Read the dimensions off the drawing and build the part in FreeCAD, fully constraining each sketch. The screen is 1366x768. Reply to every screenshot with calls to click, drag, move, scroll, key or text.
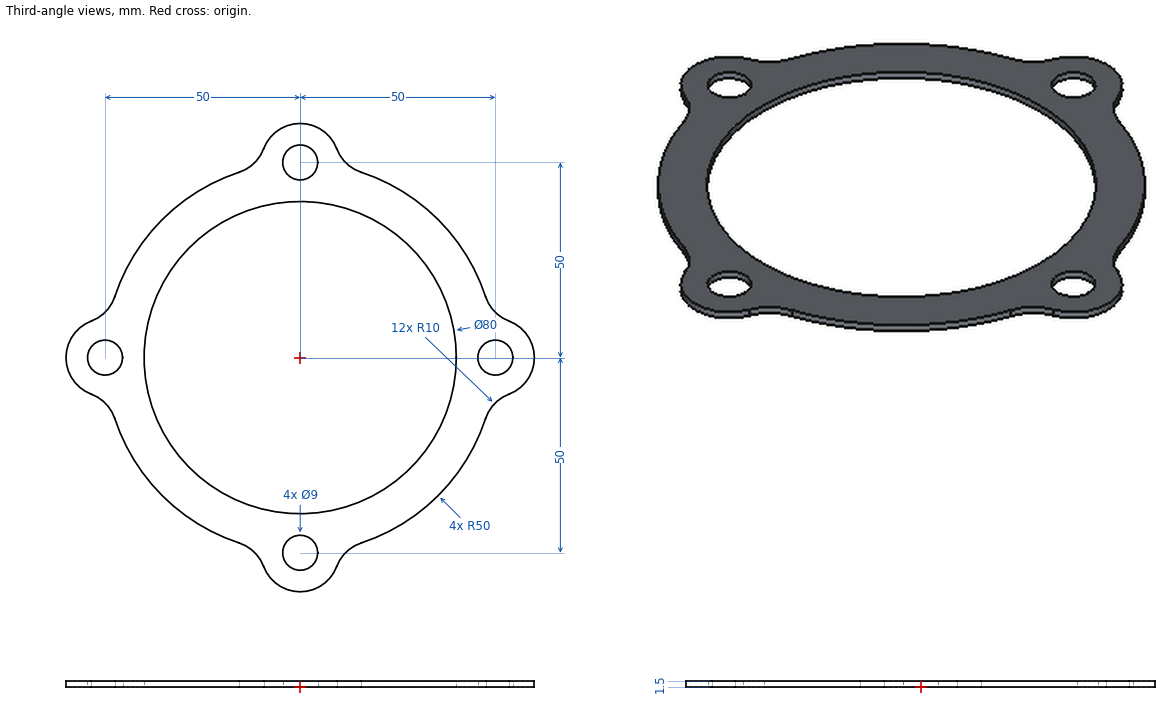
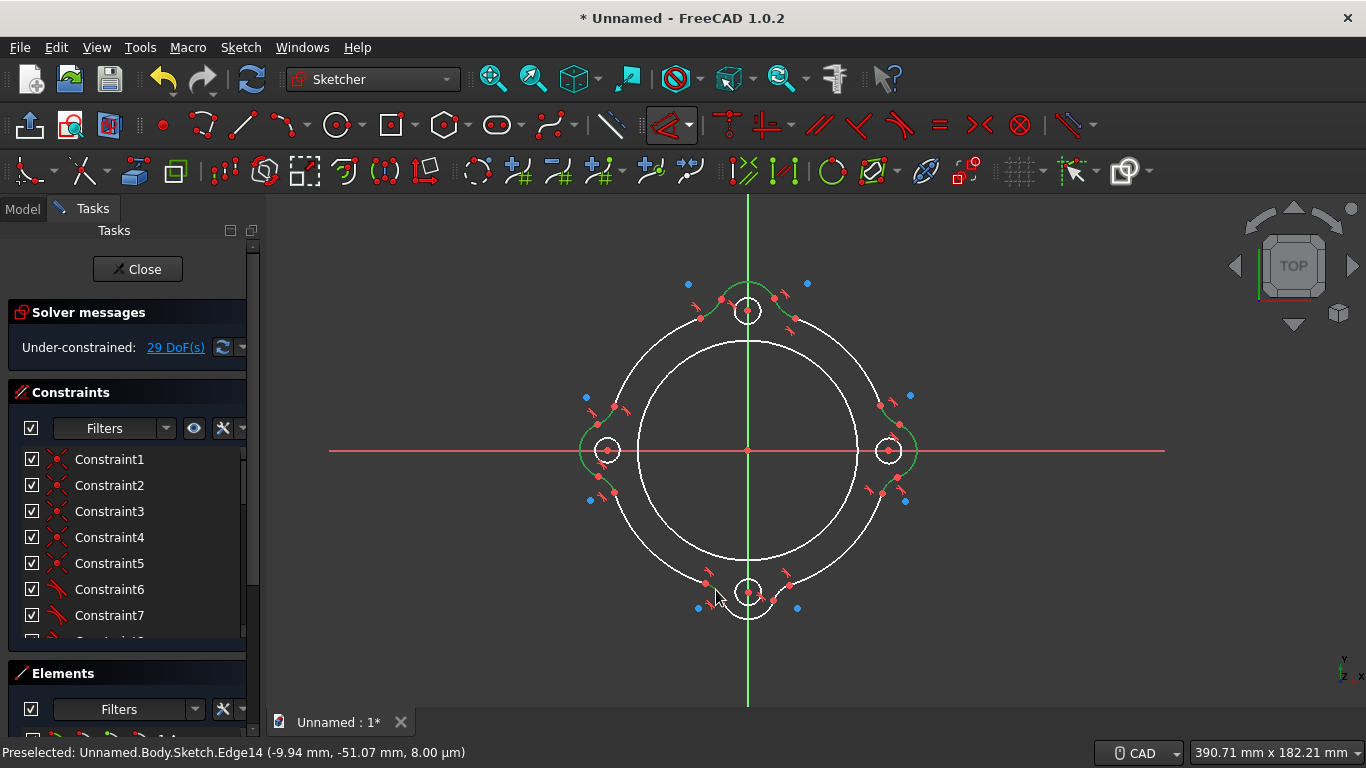
click(735, 616)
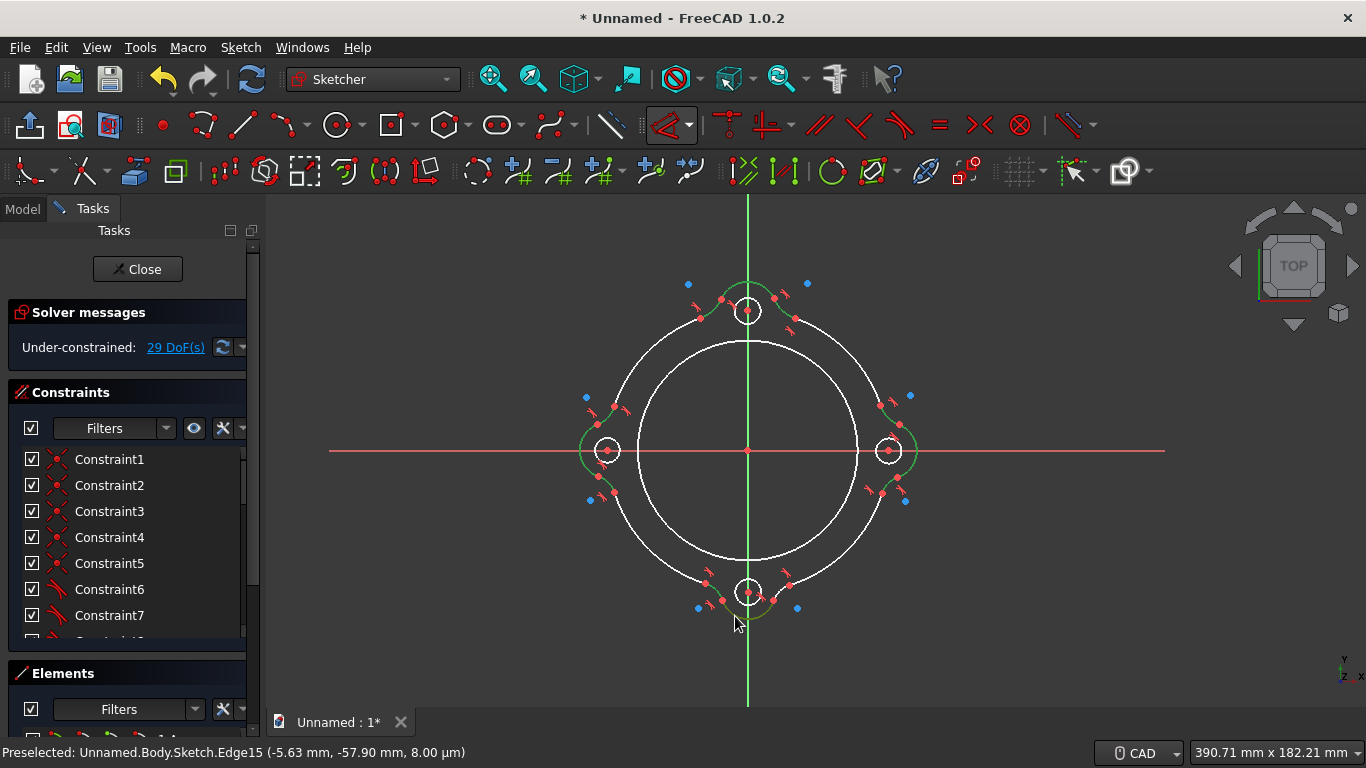
click(780, 591)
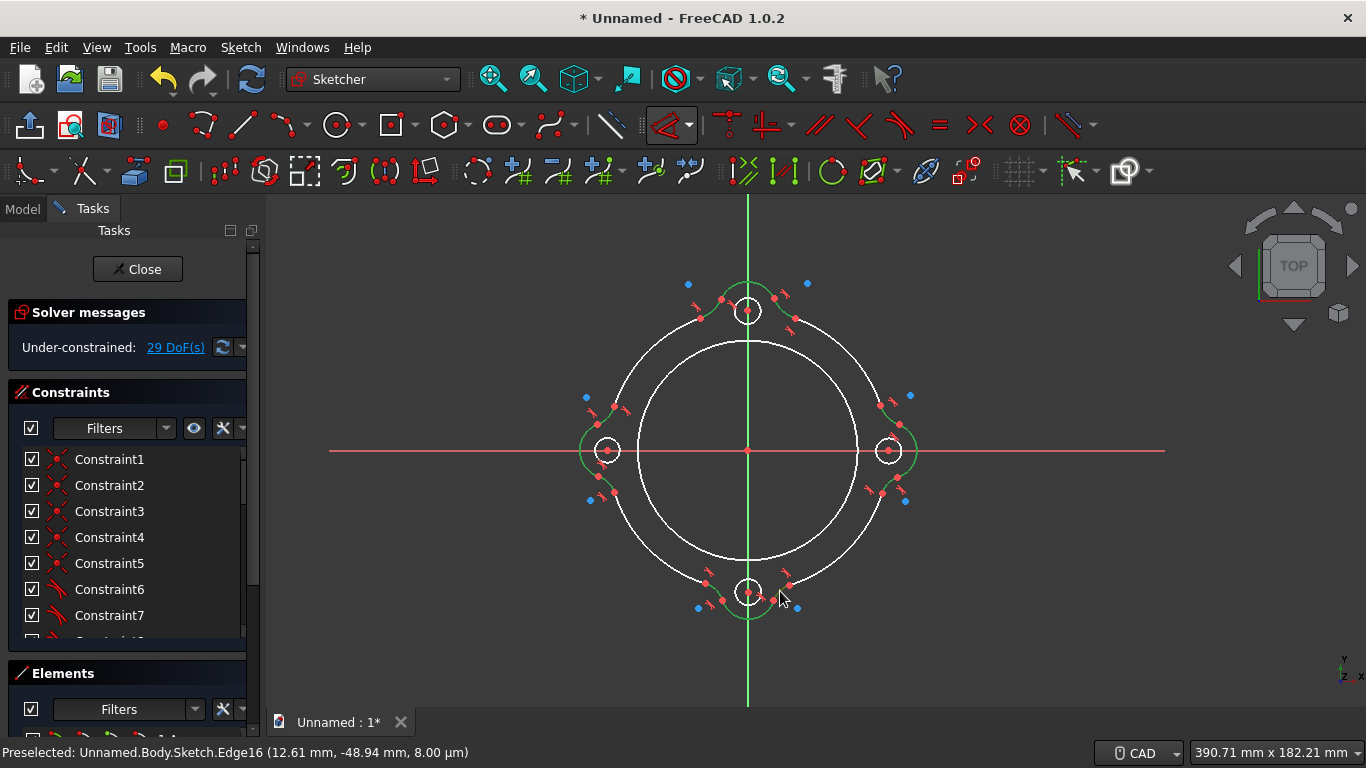
click(940, 126)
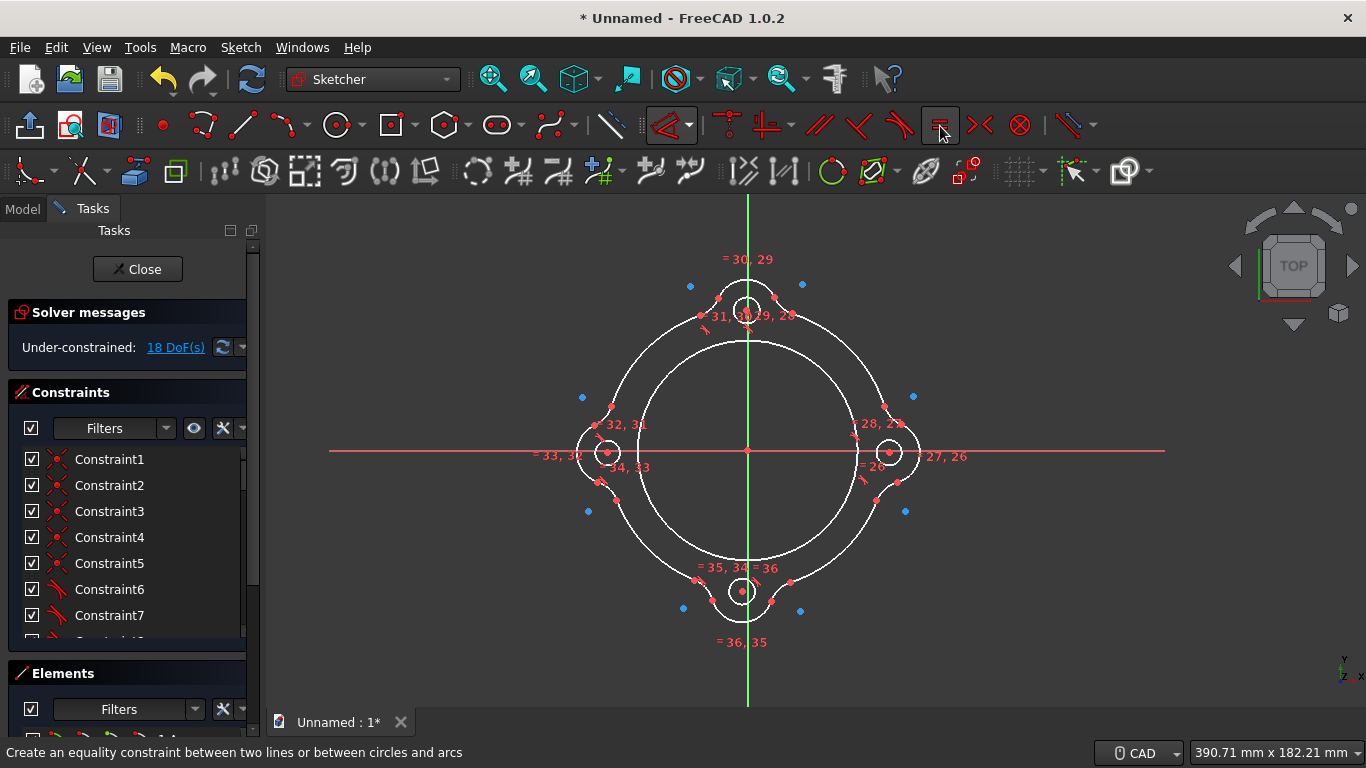
click(824, 567)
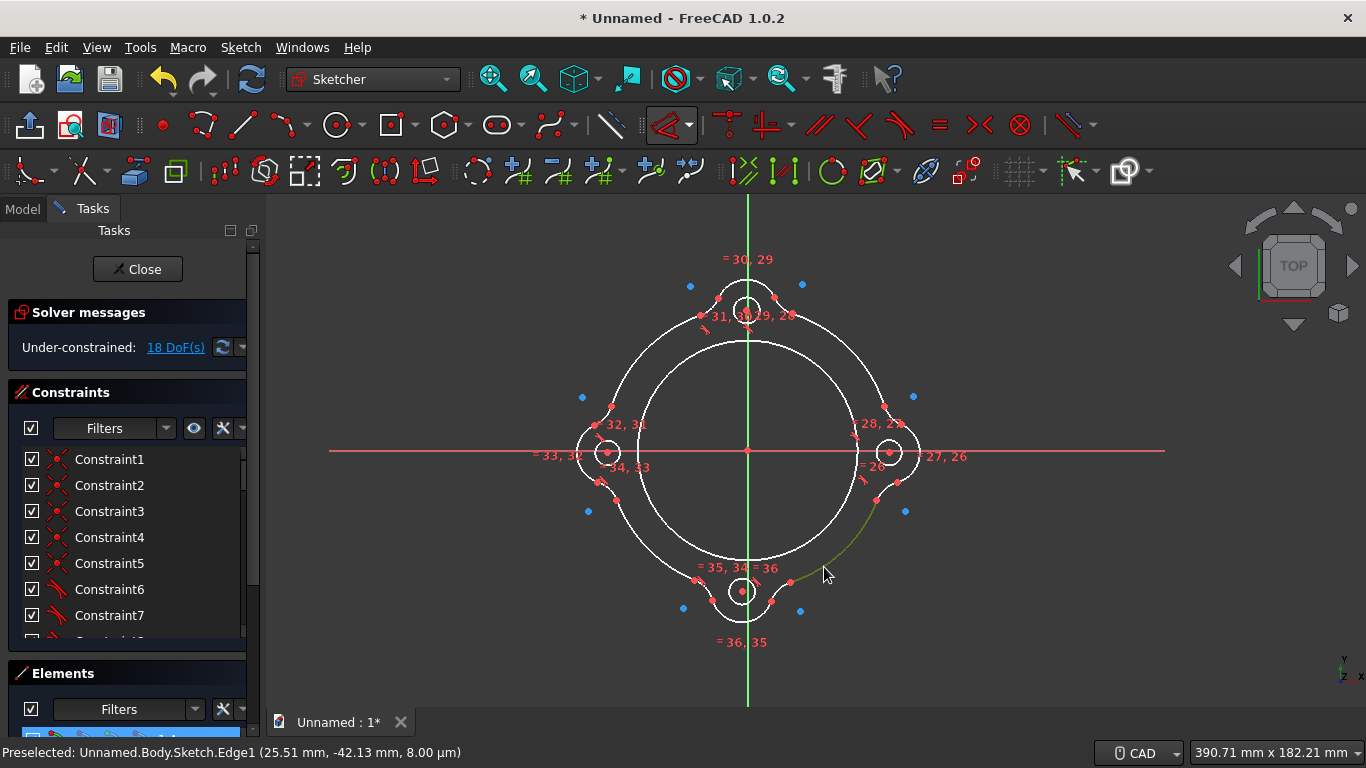
click(867, 370)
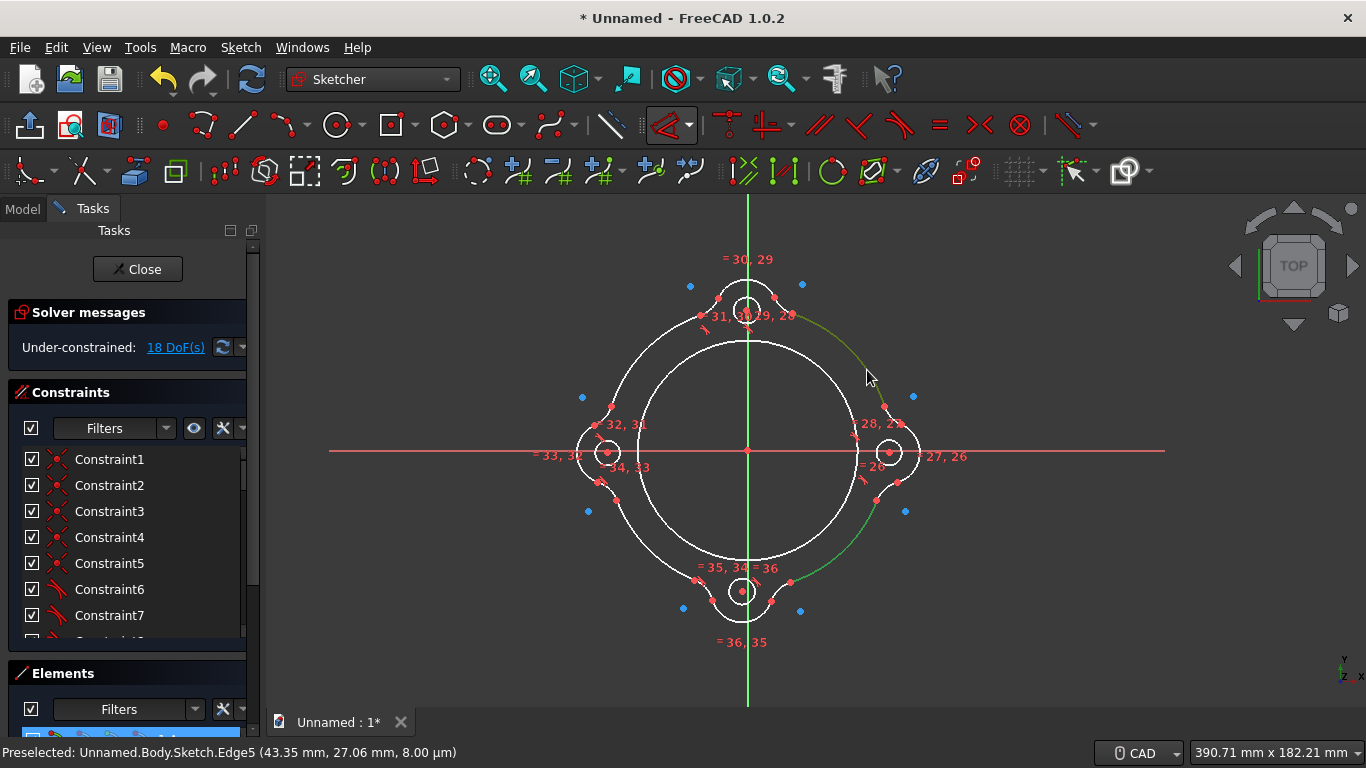
click(665, 333)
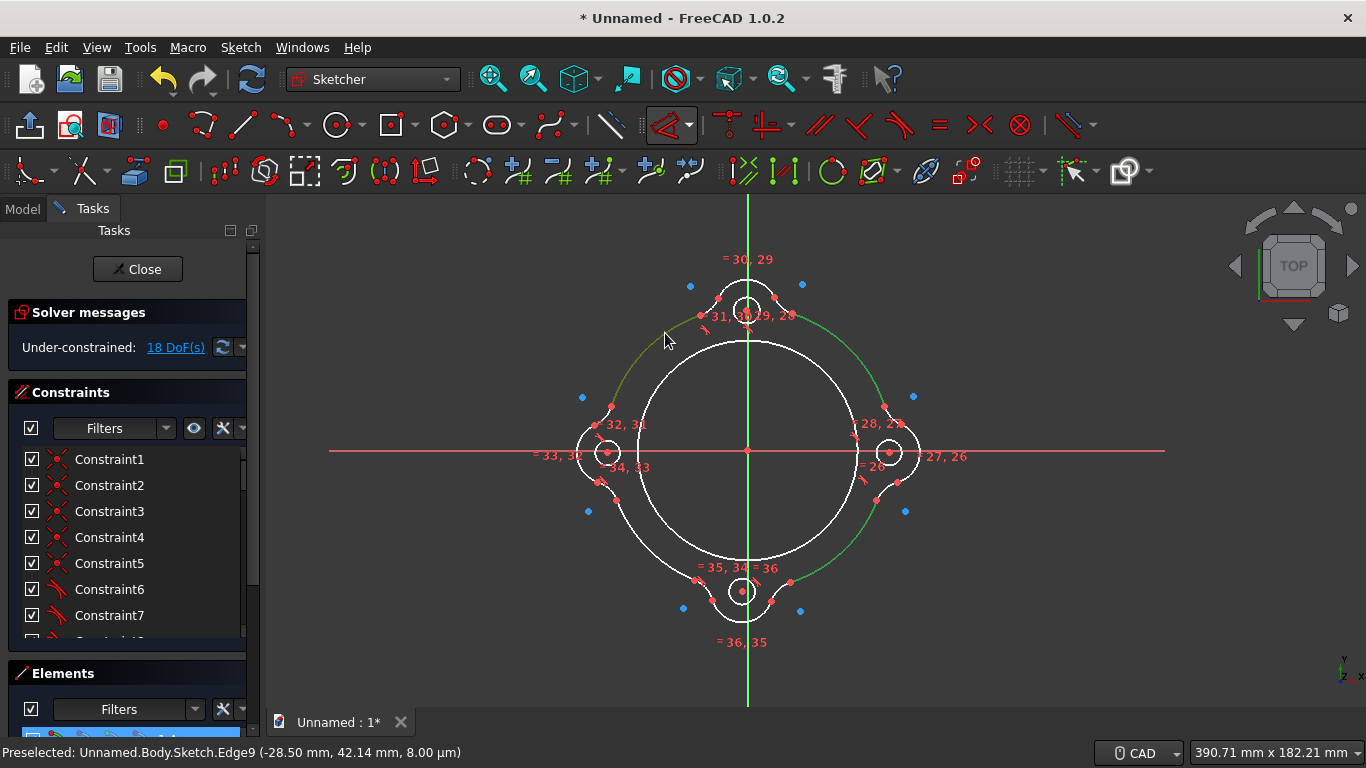
click(633, 531)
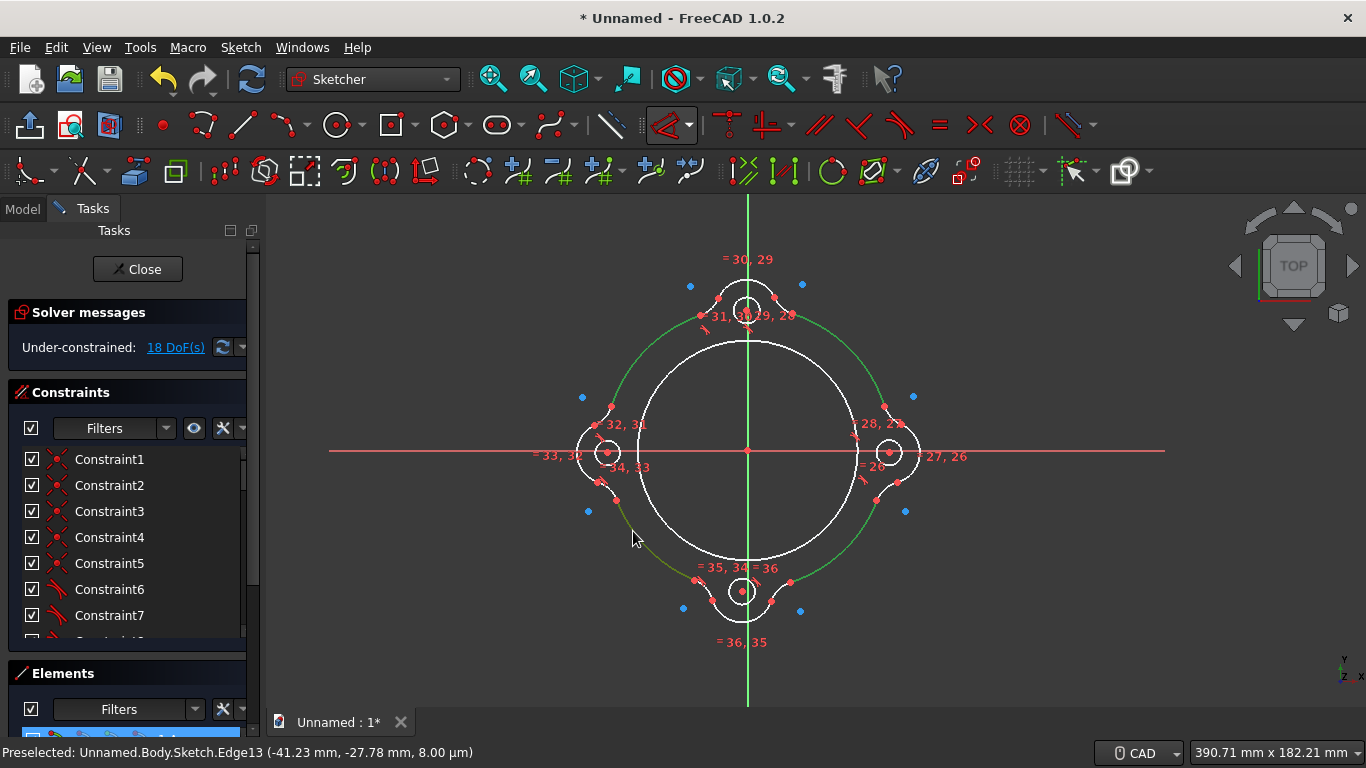
click(940, 126)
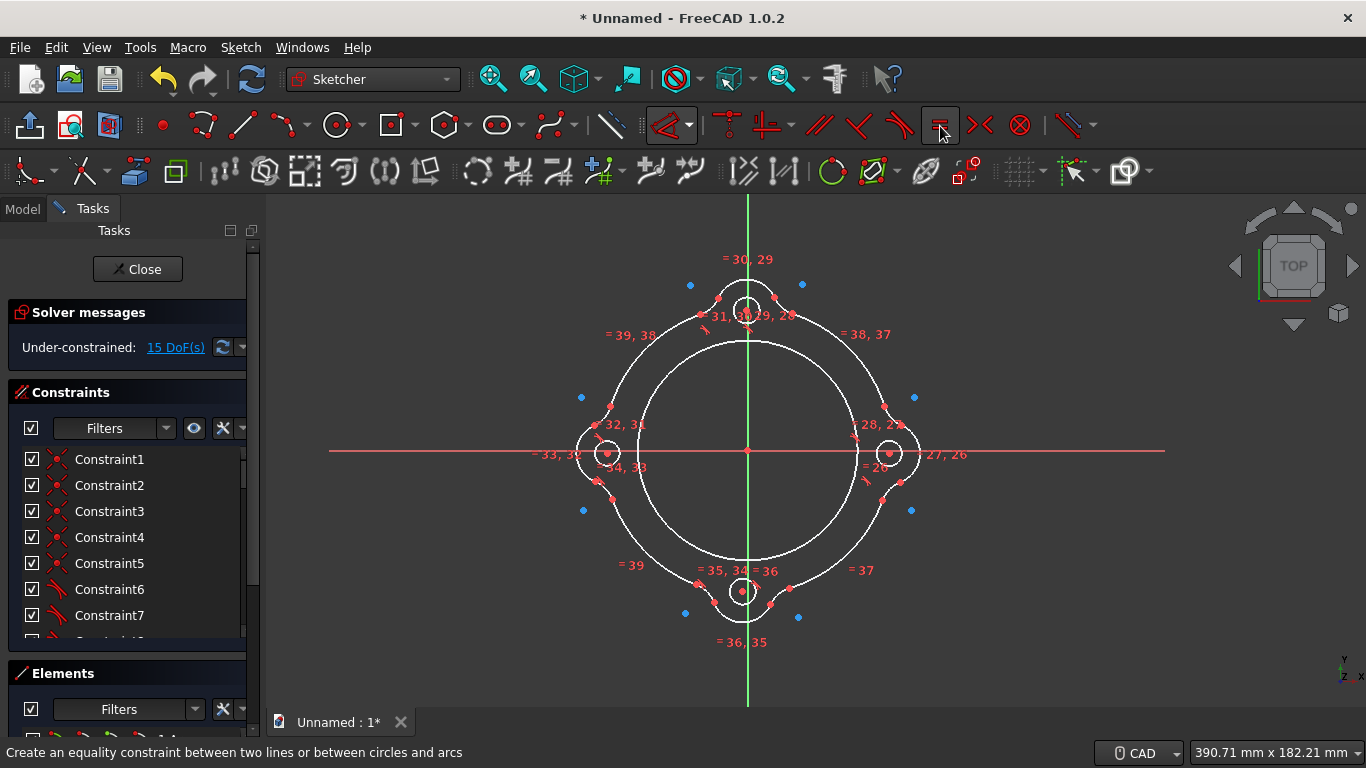
click(734, 601)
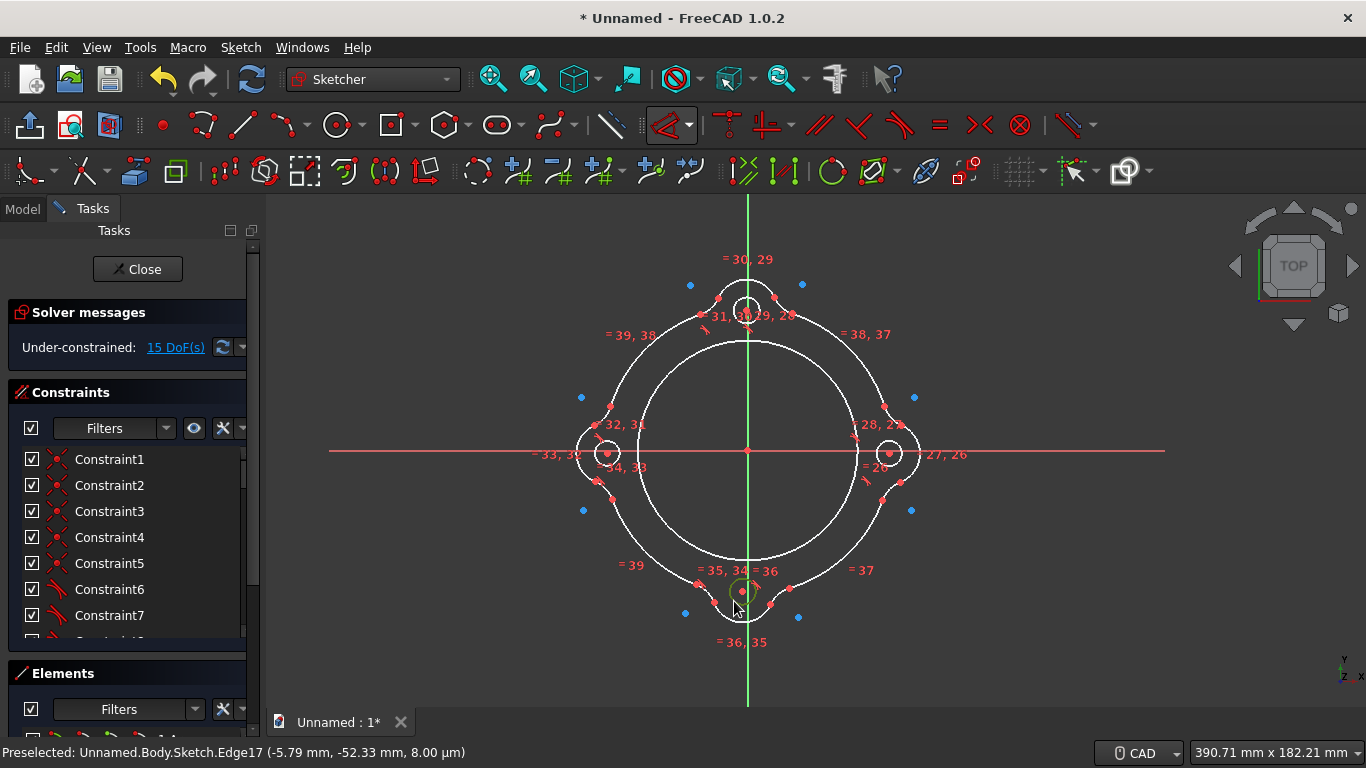
click(595, 453)